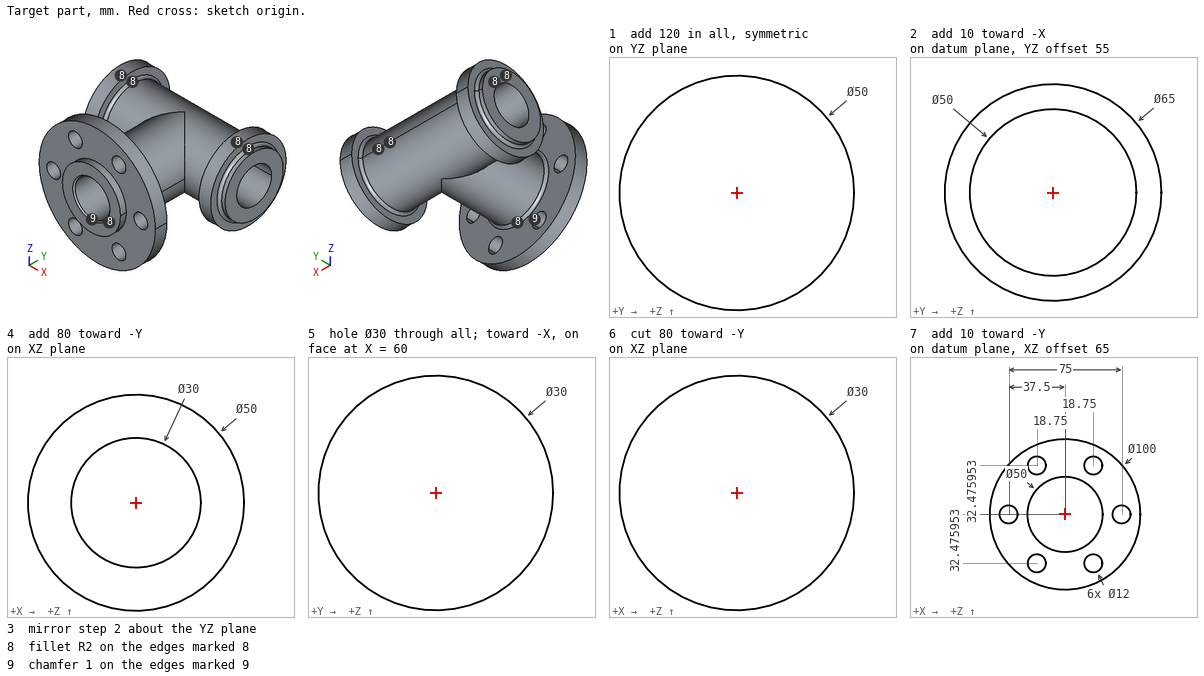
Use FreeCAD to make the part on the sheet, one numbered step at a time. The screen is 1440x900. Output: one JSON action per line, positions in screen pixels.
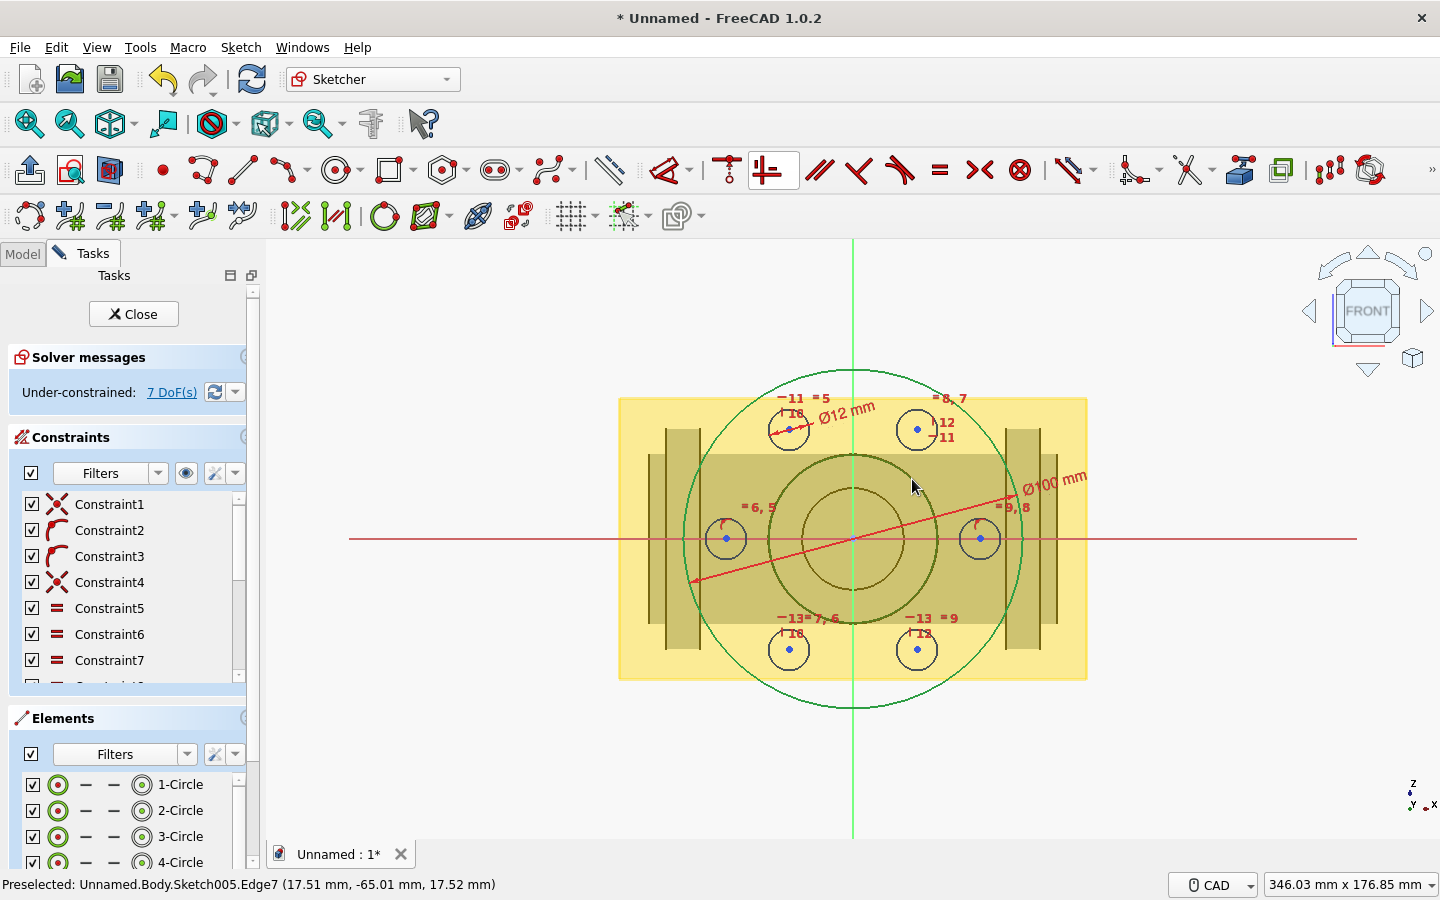
{"action": "key", "text": "k o"}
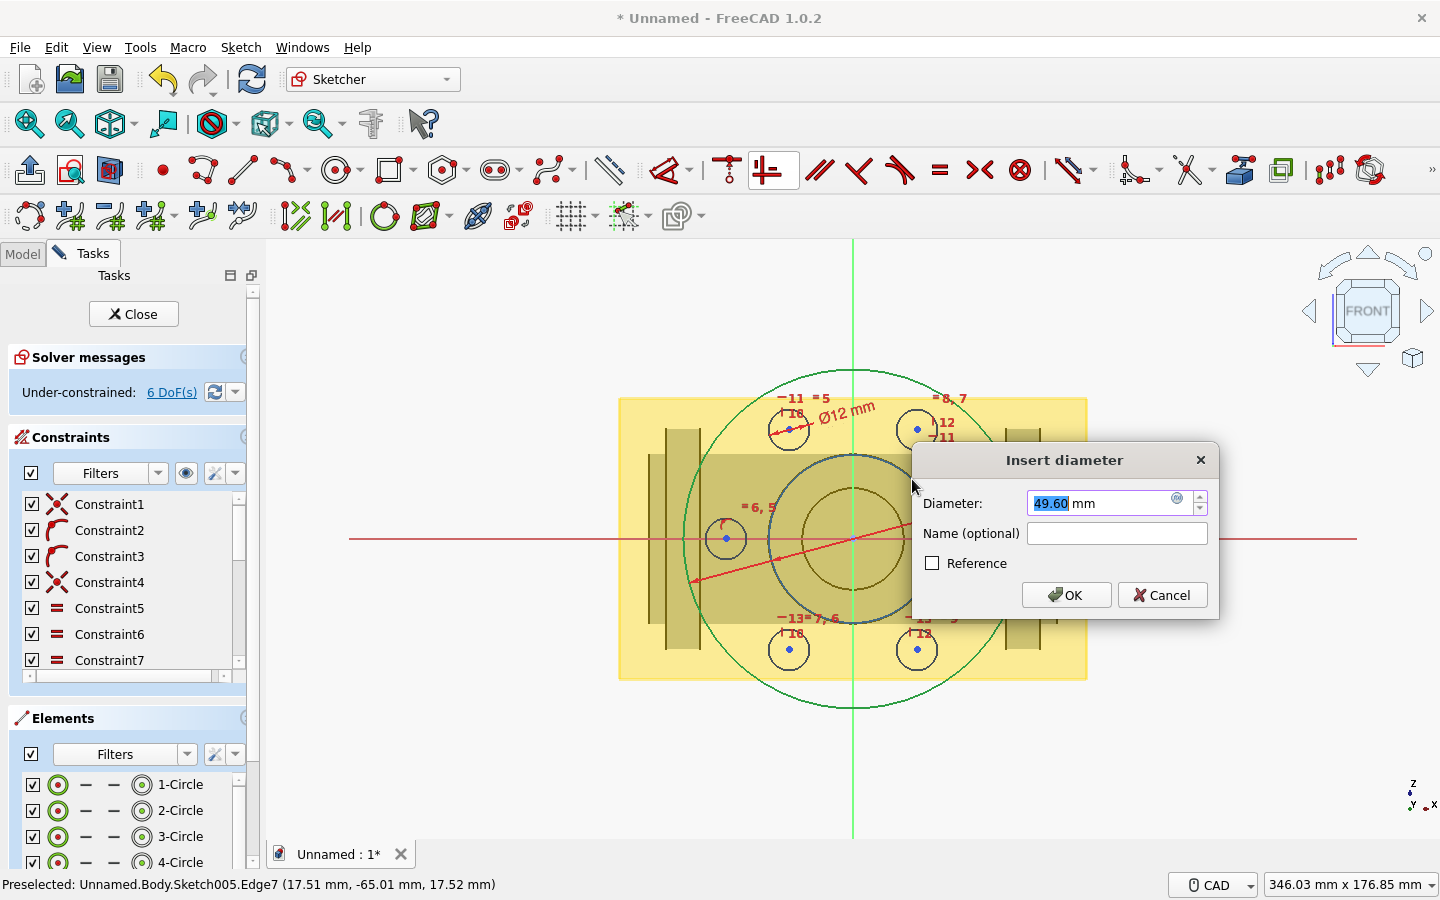
{"action": "type", "text": "50"}
{"action": "key", "text": "Return"}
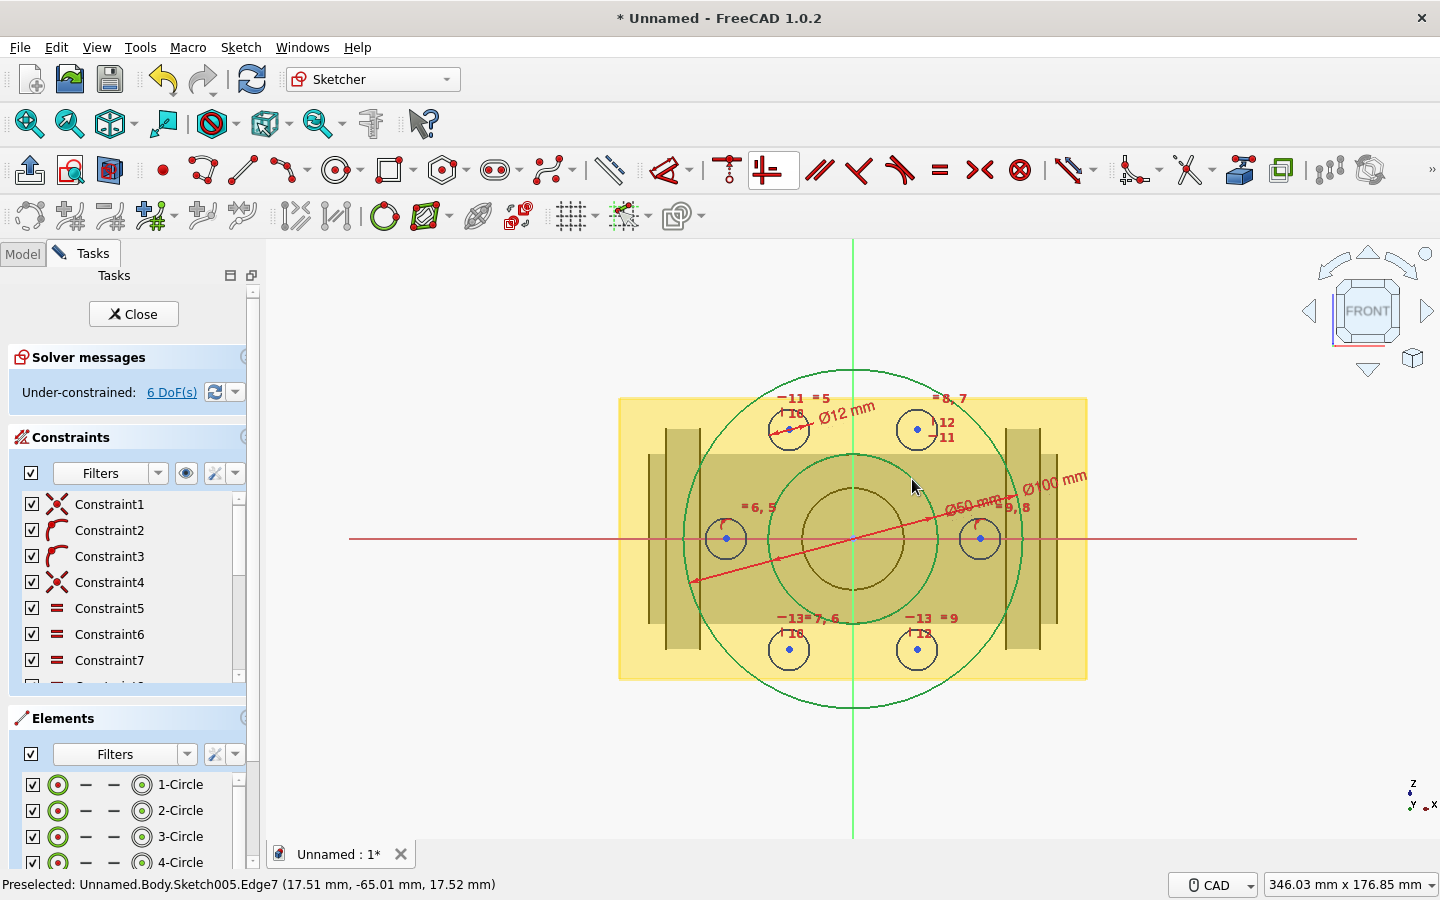
{"action": "left_click", "coordinate": [726, 539]}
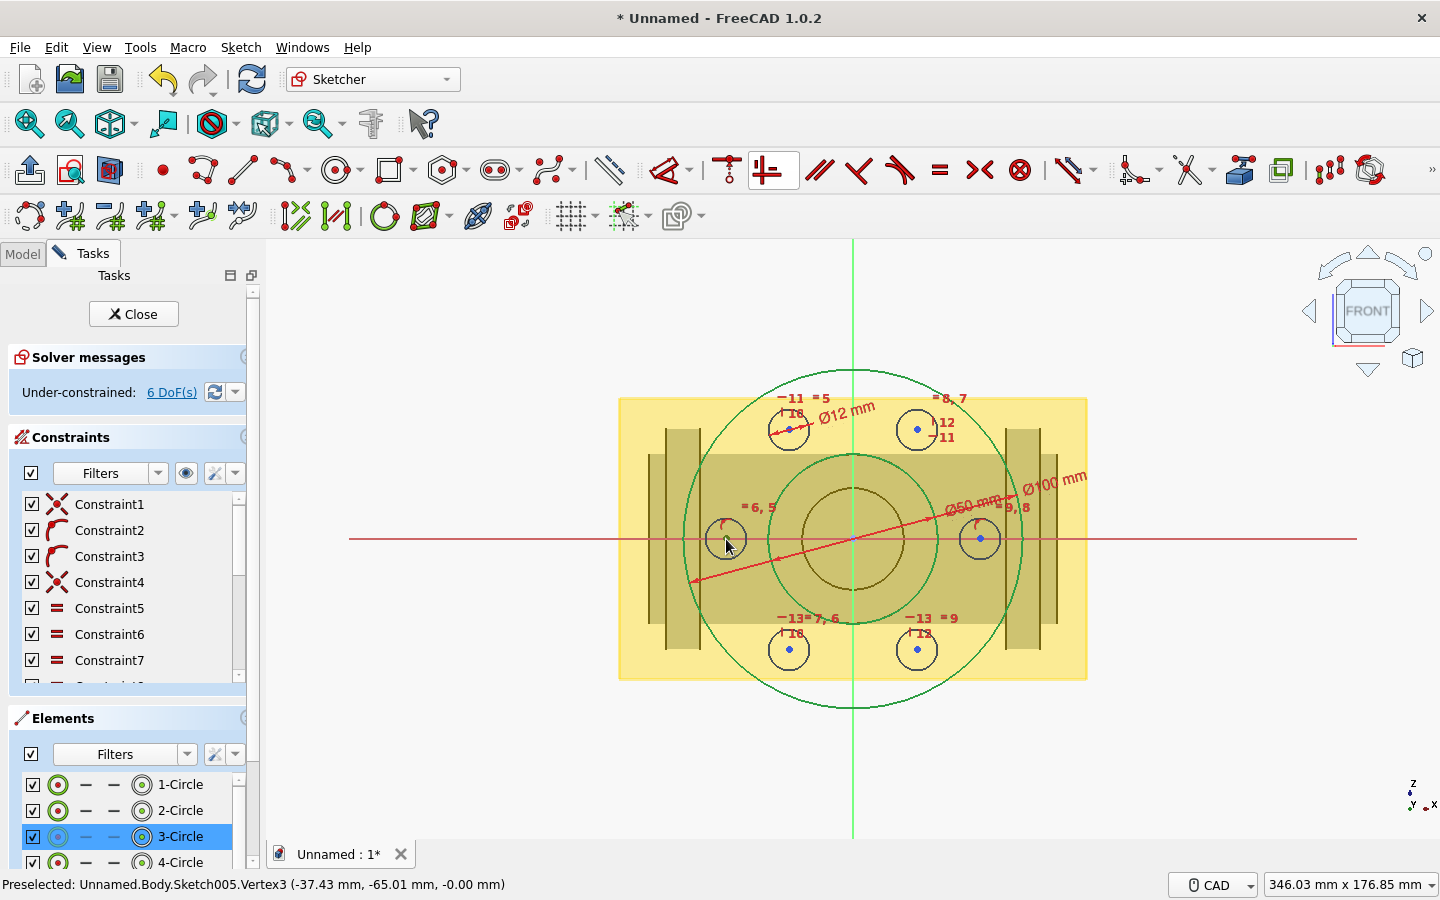
{"action": "left_click", "coordinate": [980, 539]}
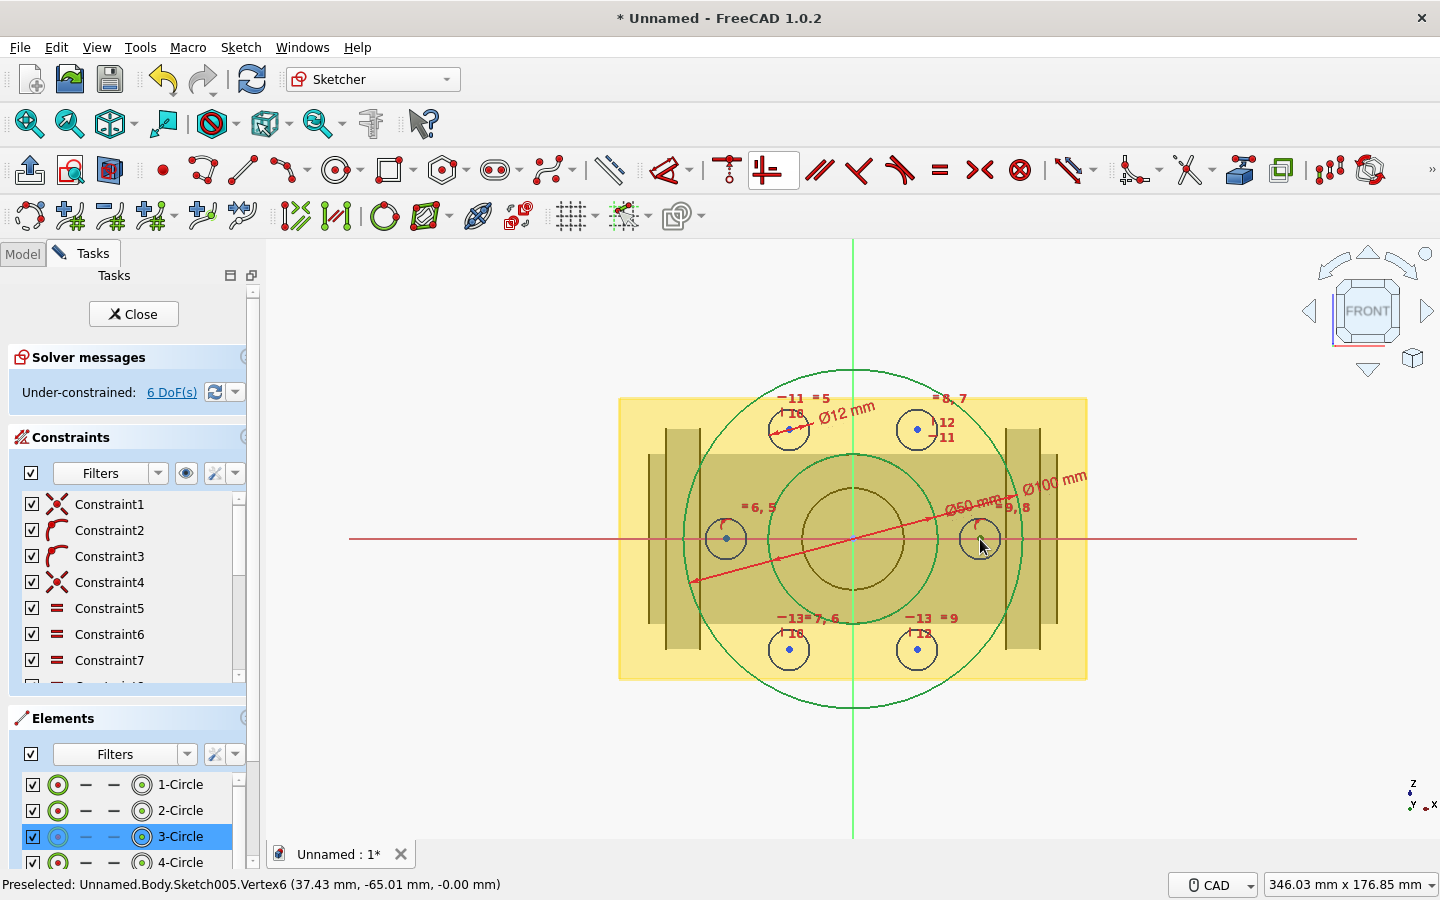
{"action": "key", "text": "l"}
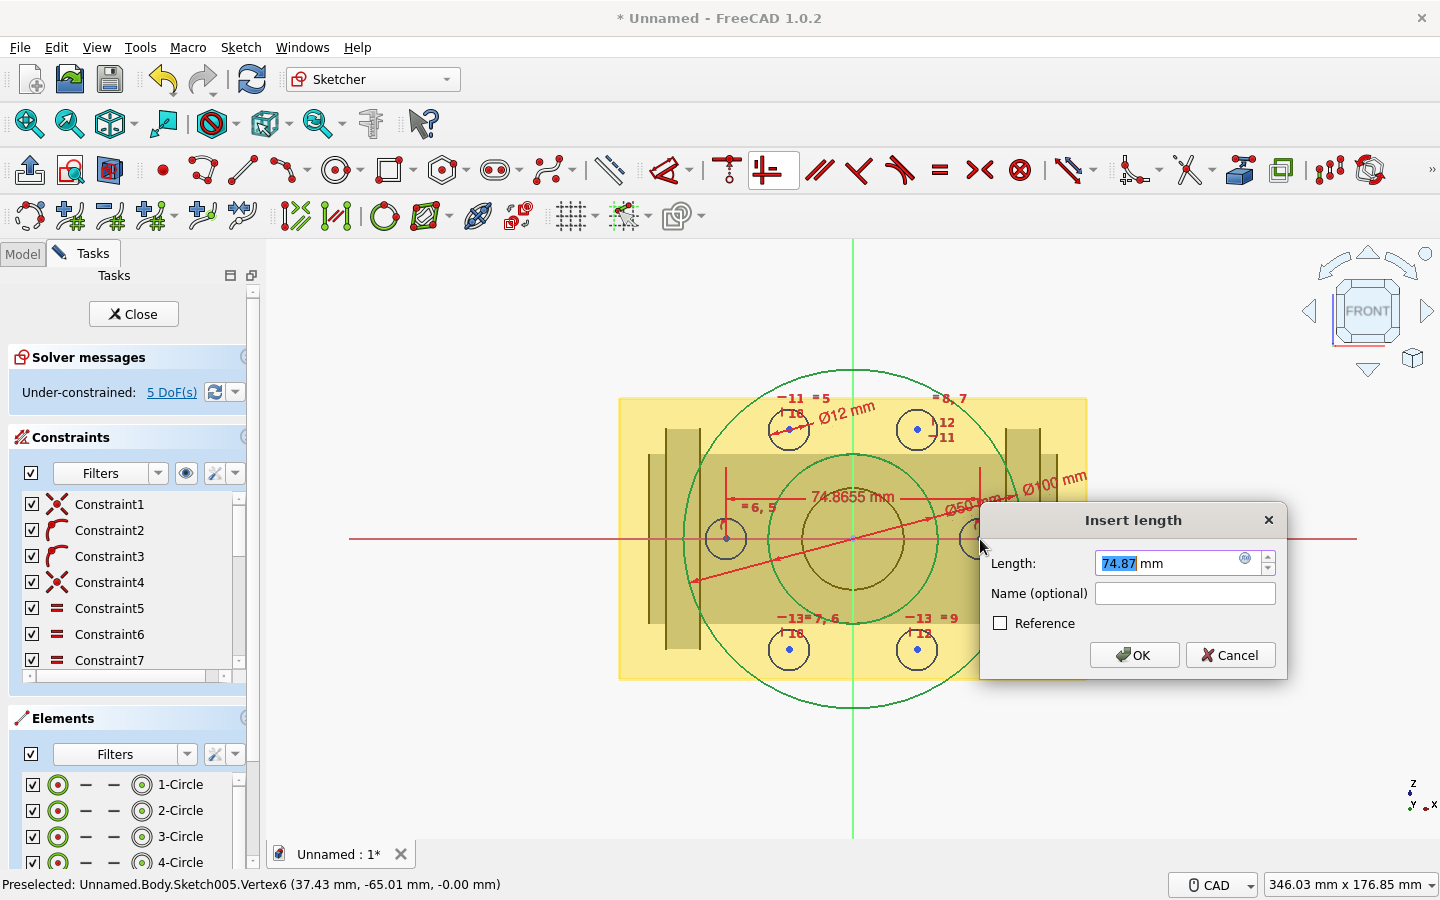
{"action": "type", "text": "75"}
{"action": "key", "text": "Return"}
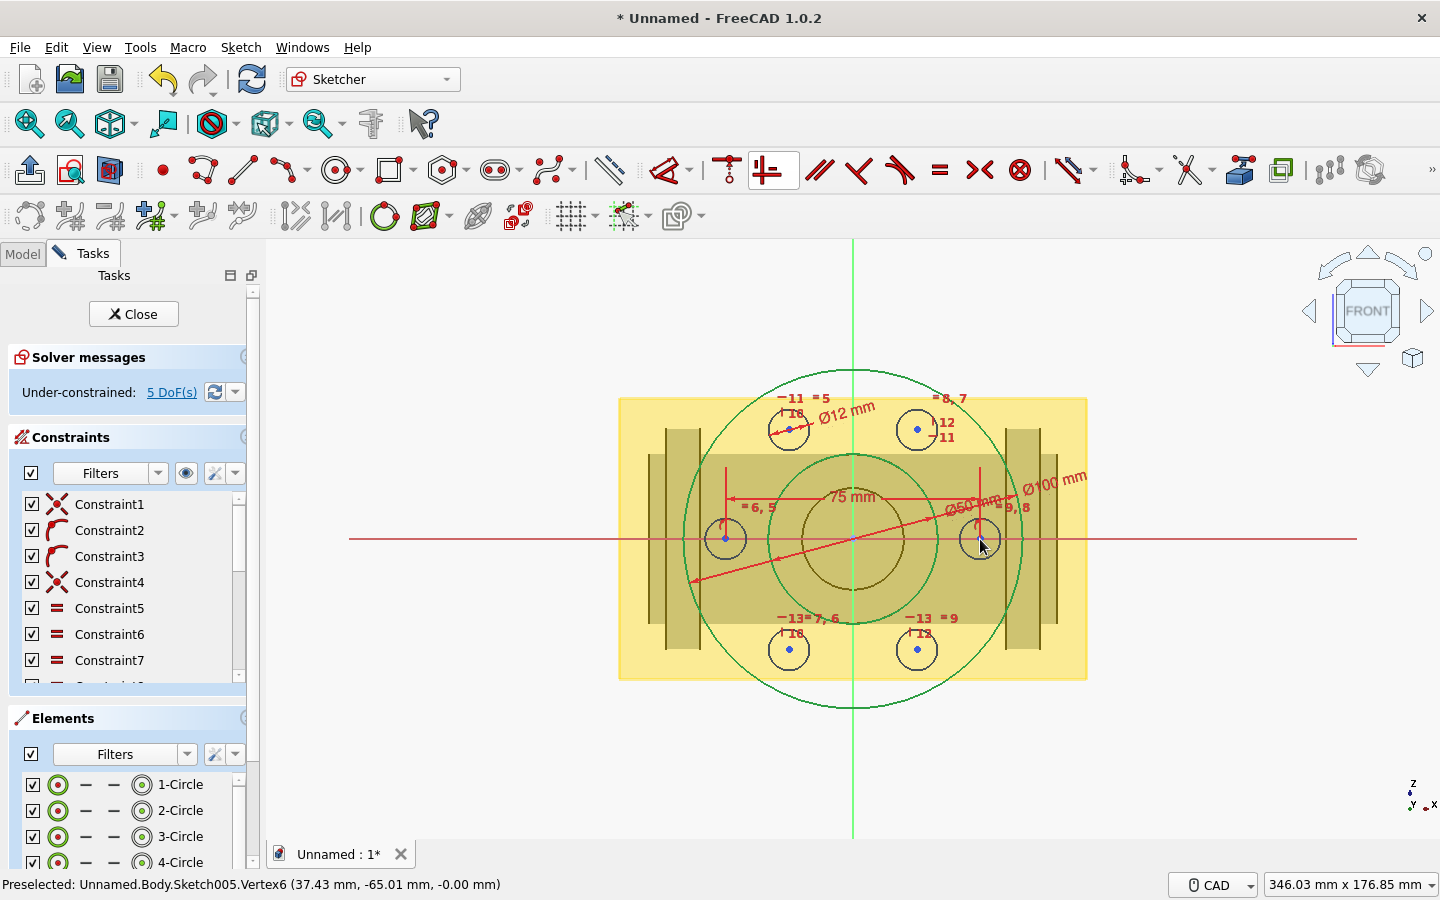
{"action": "left_click", "coordinate": [726, 539]}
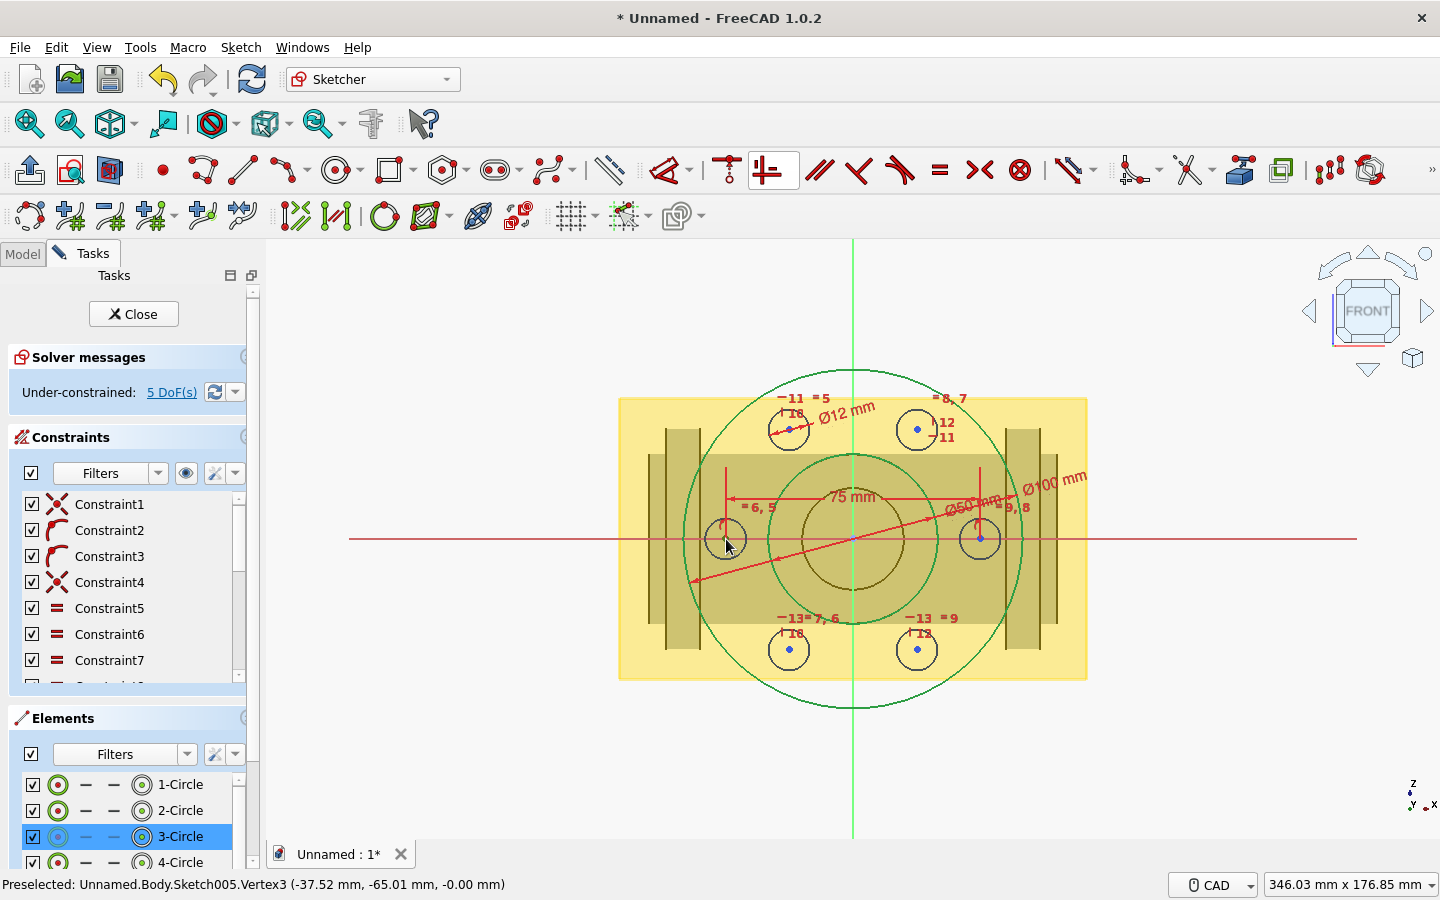
{"action": "key", "text": "l"}